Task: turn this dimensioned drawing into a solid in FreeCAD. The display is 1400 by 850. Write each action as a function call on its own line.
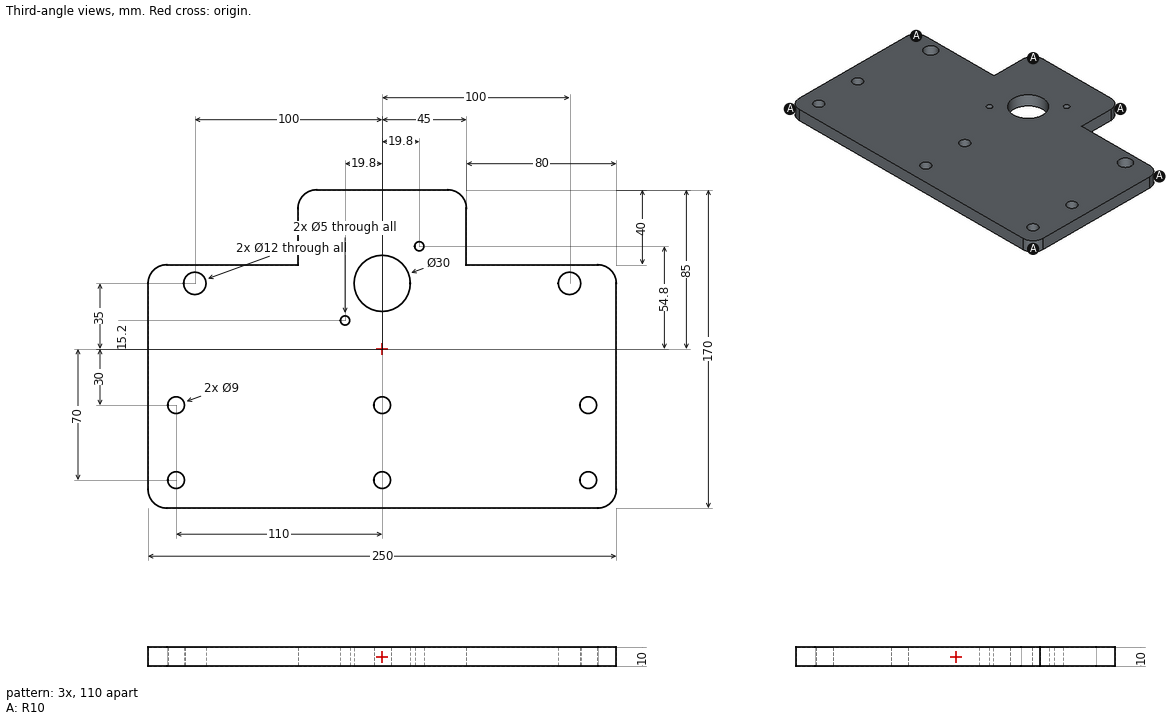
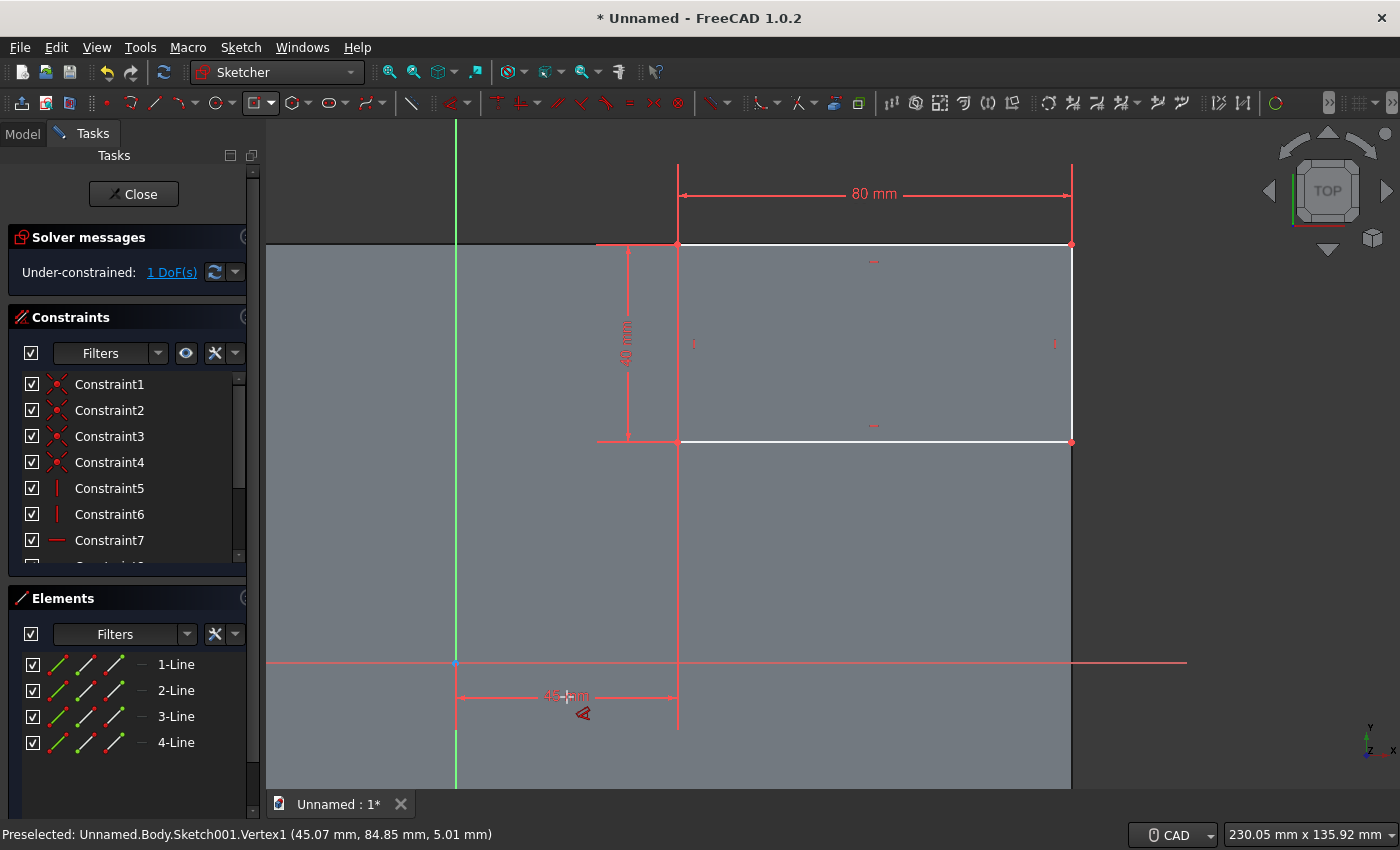
click(678, 245)
click(422, 454)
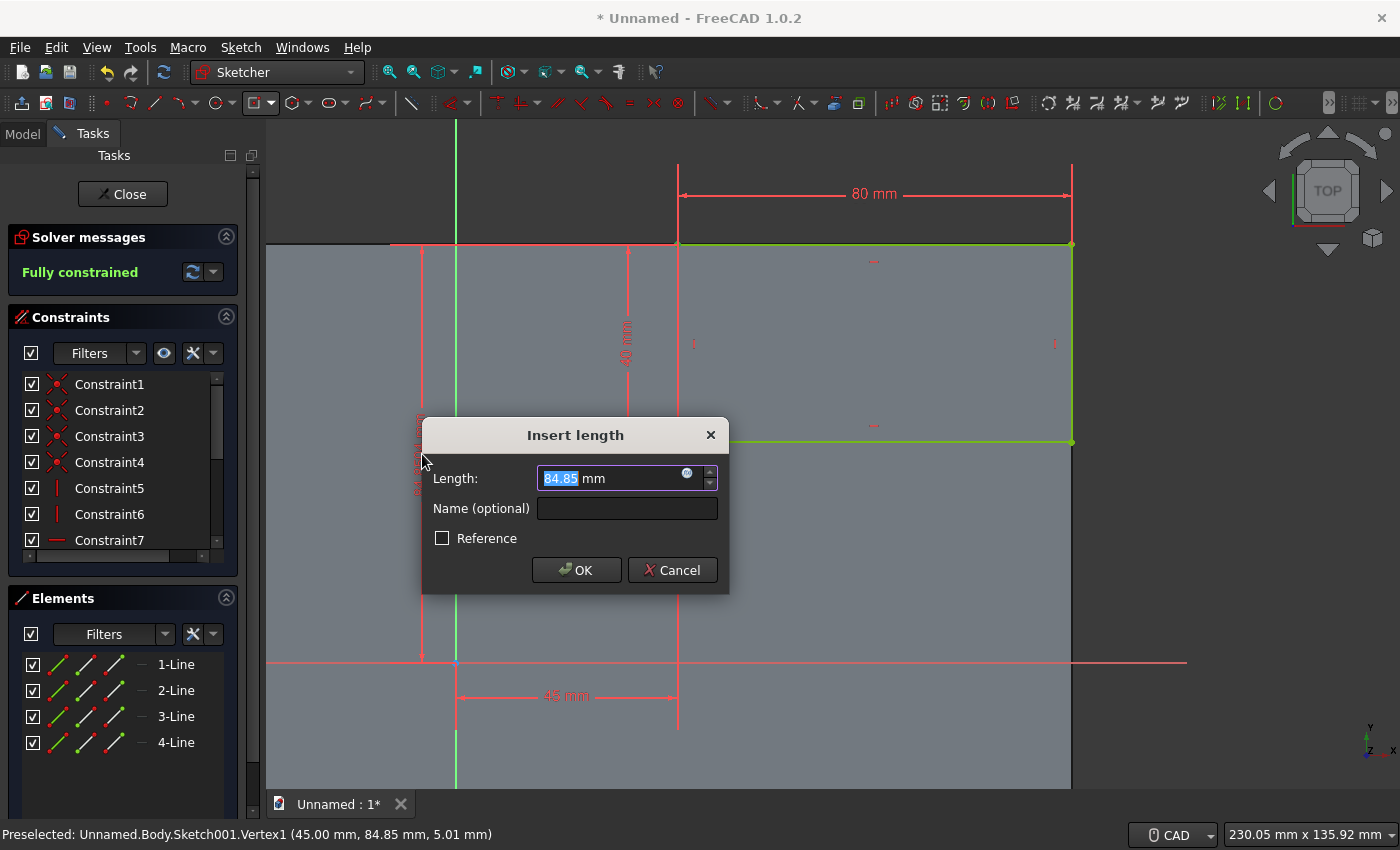
text(85)
key(Return)
key(Escape)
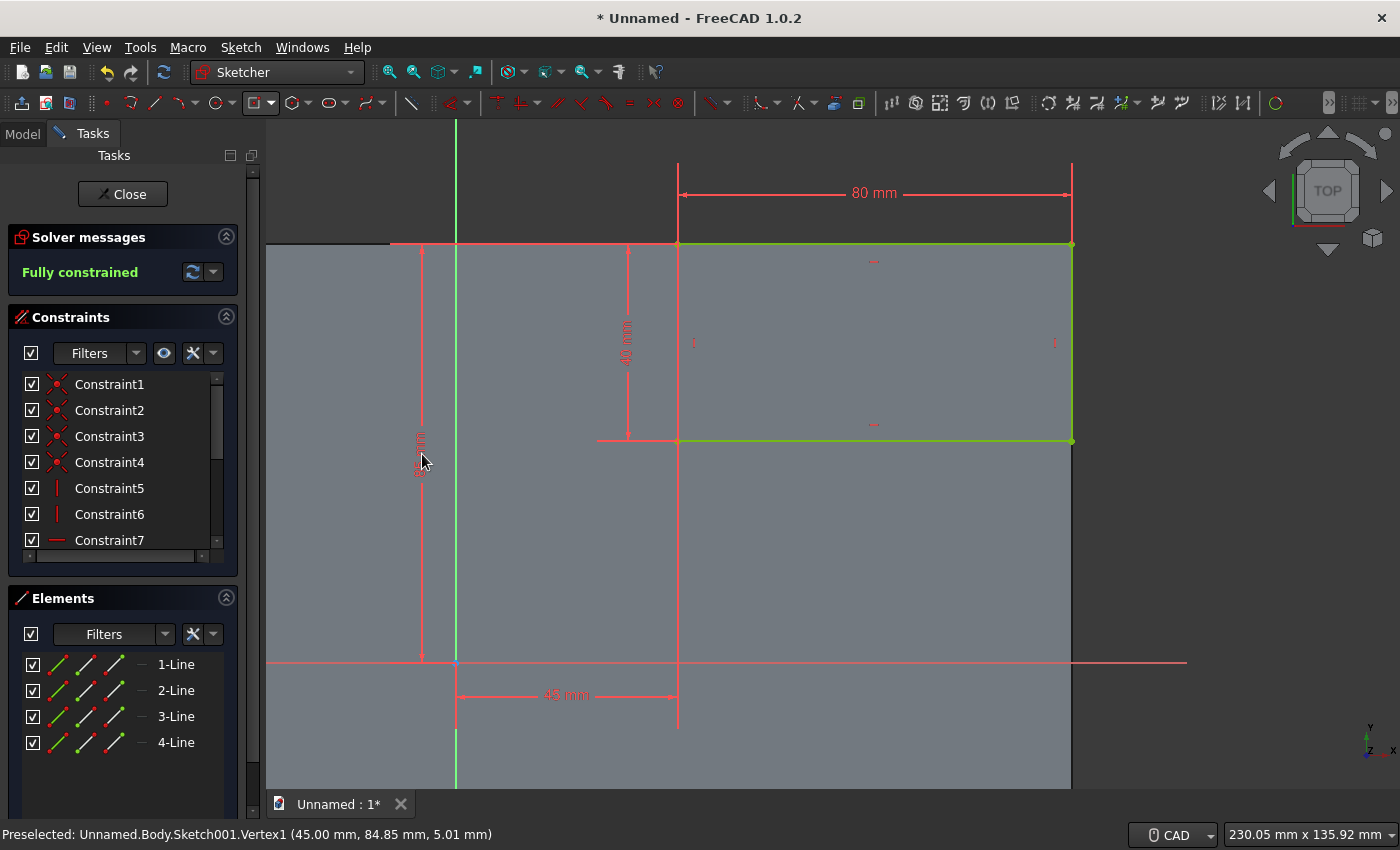
click(123, 194)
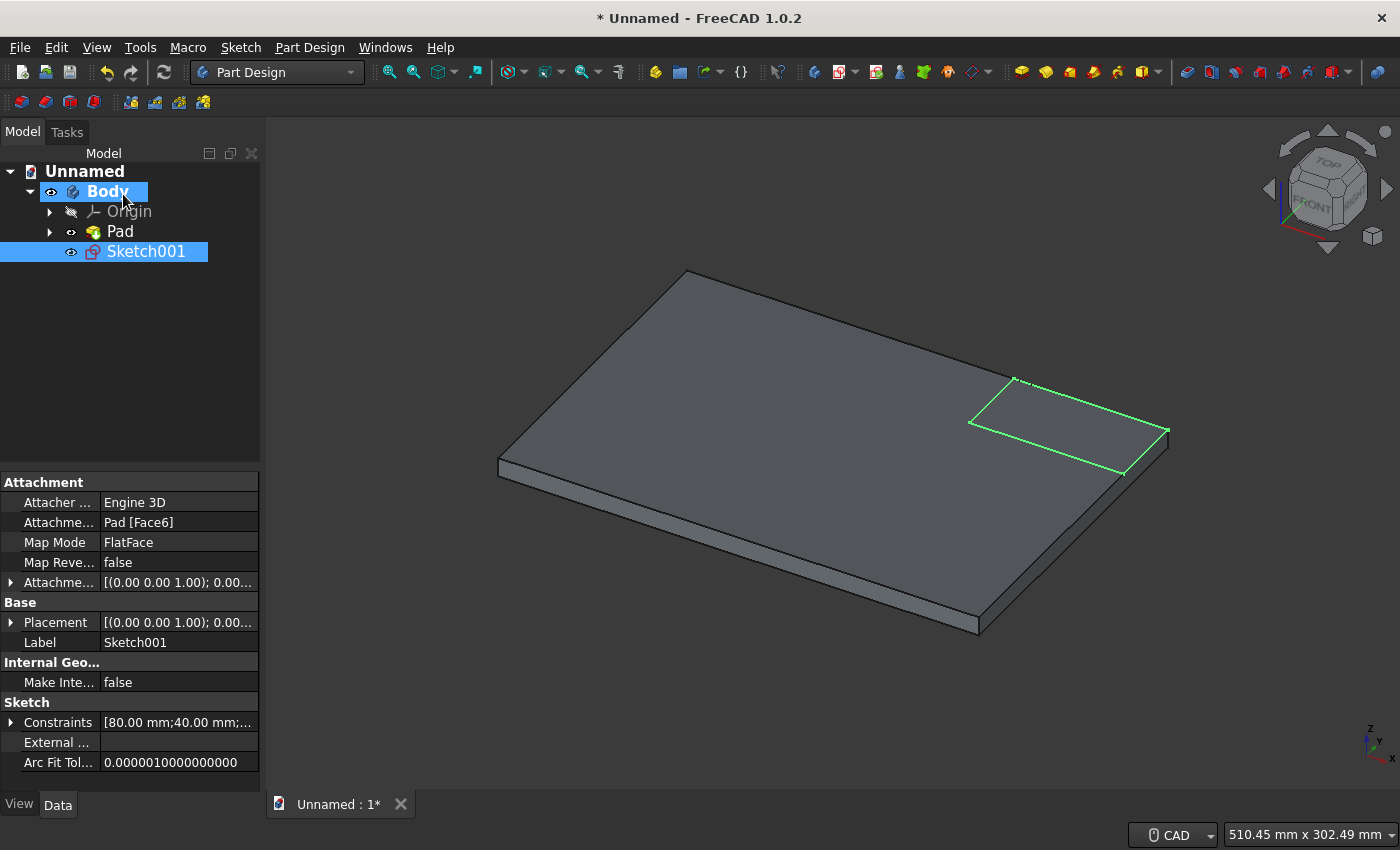
click(1188, 72)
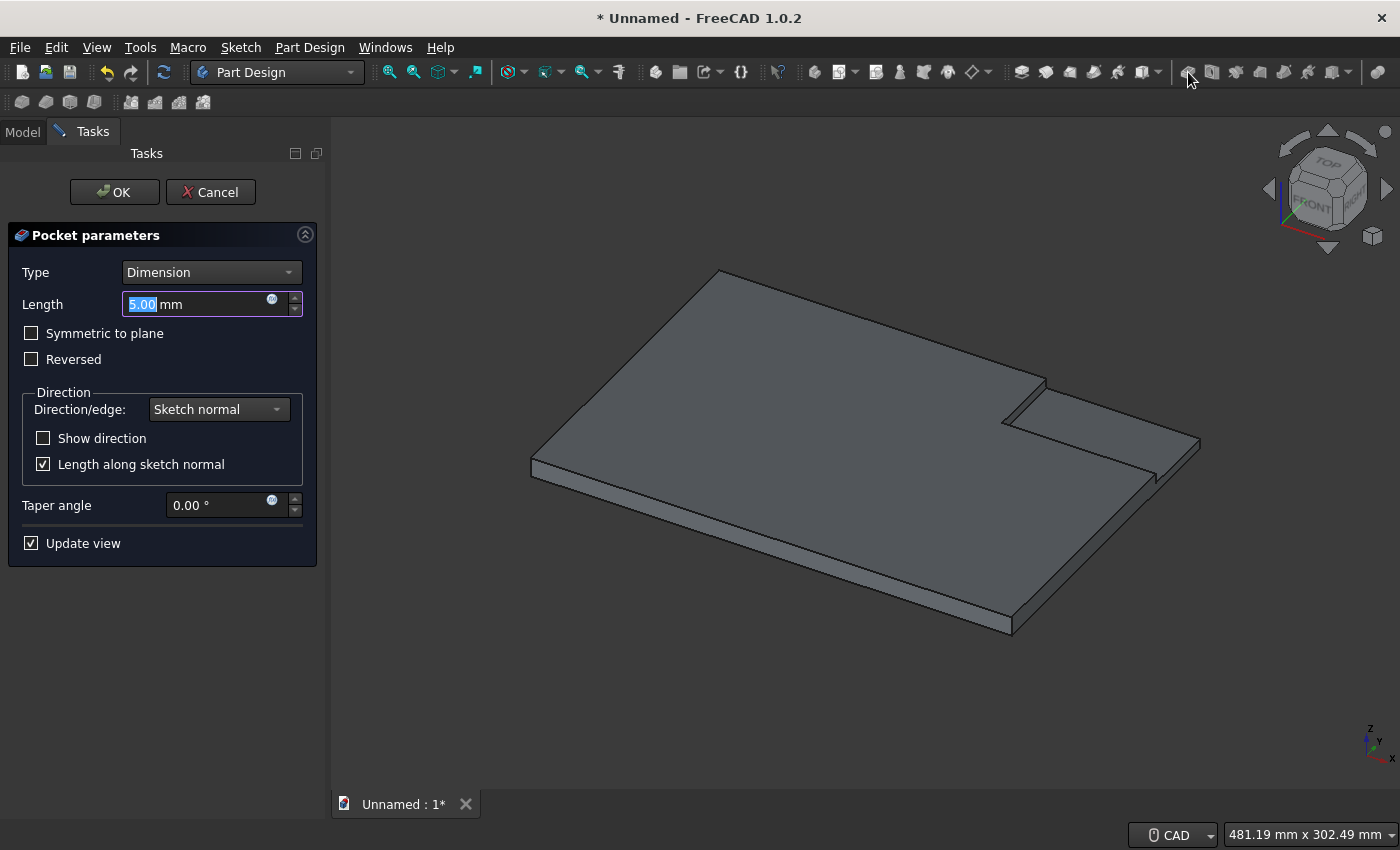
text(10)
key(Tab)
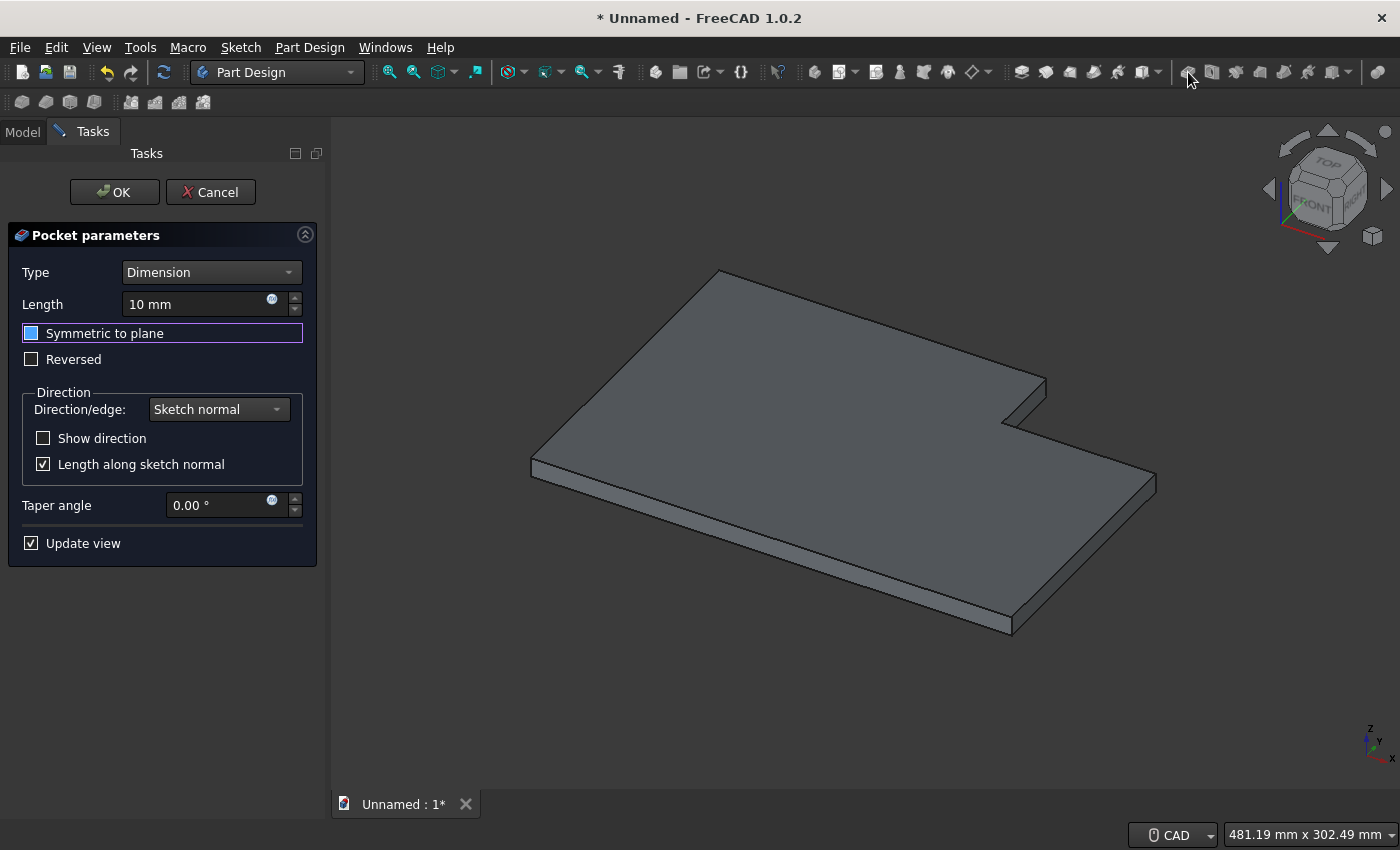
click(115, 192)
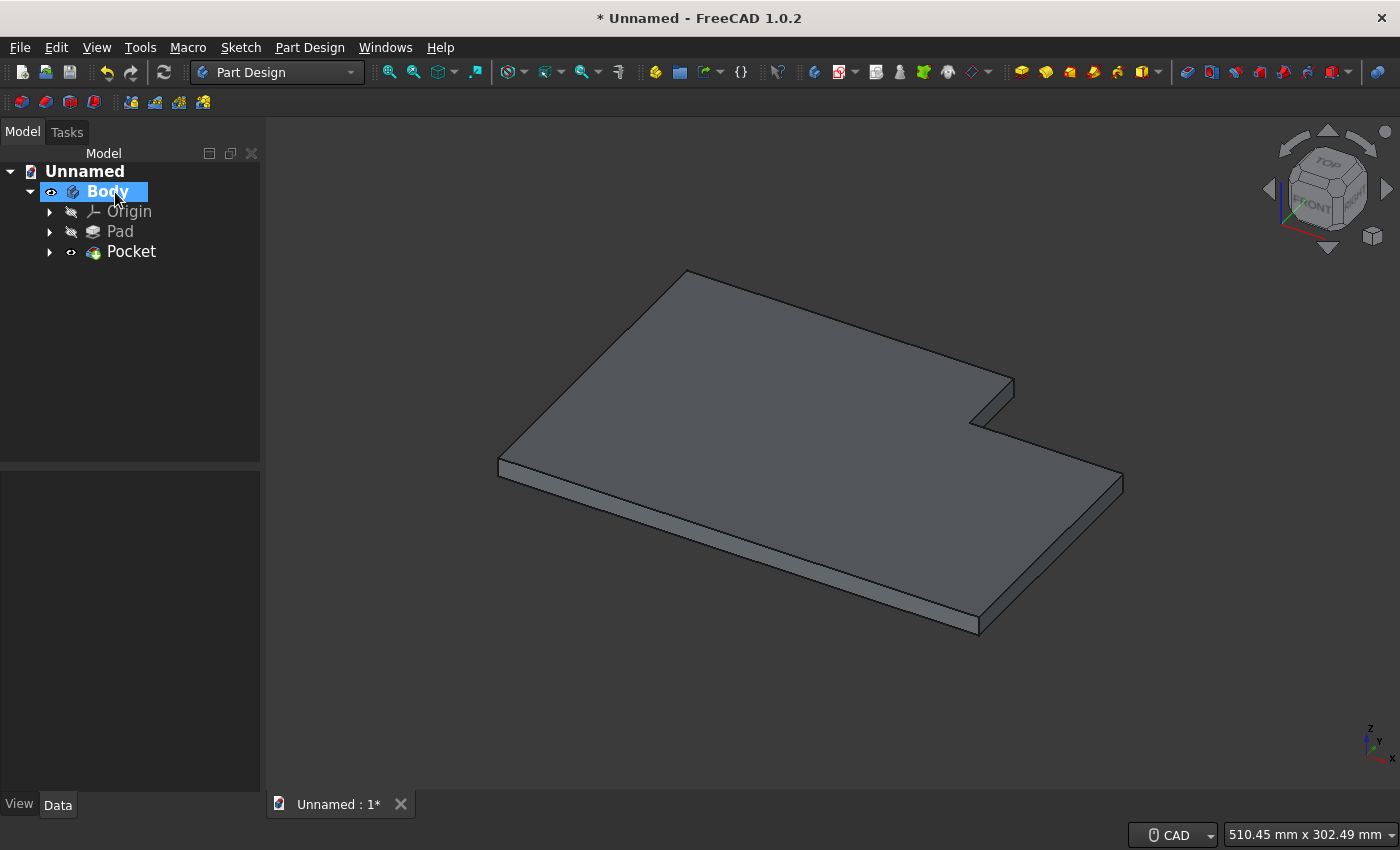
click(116, 252)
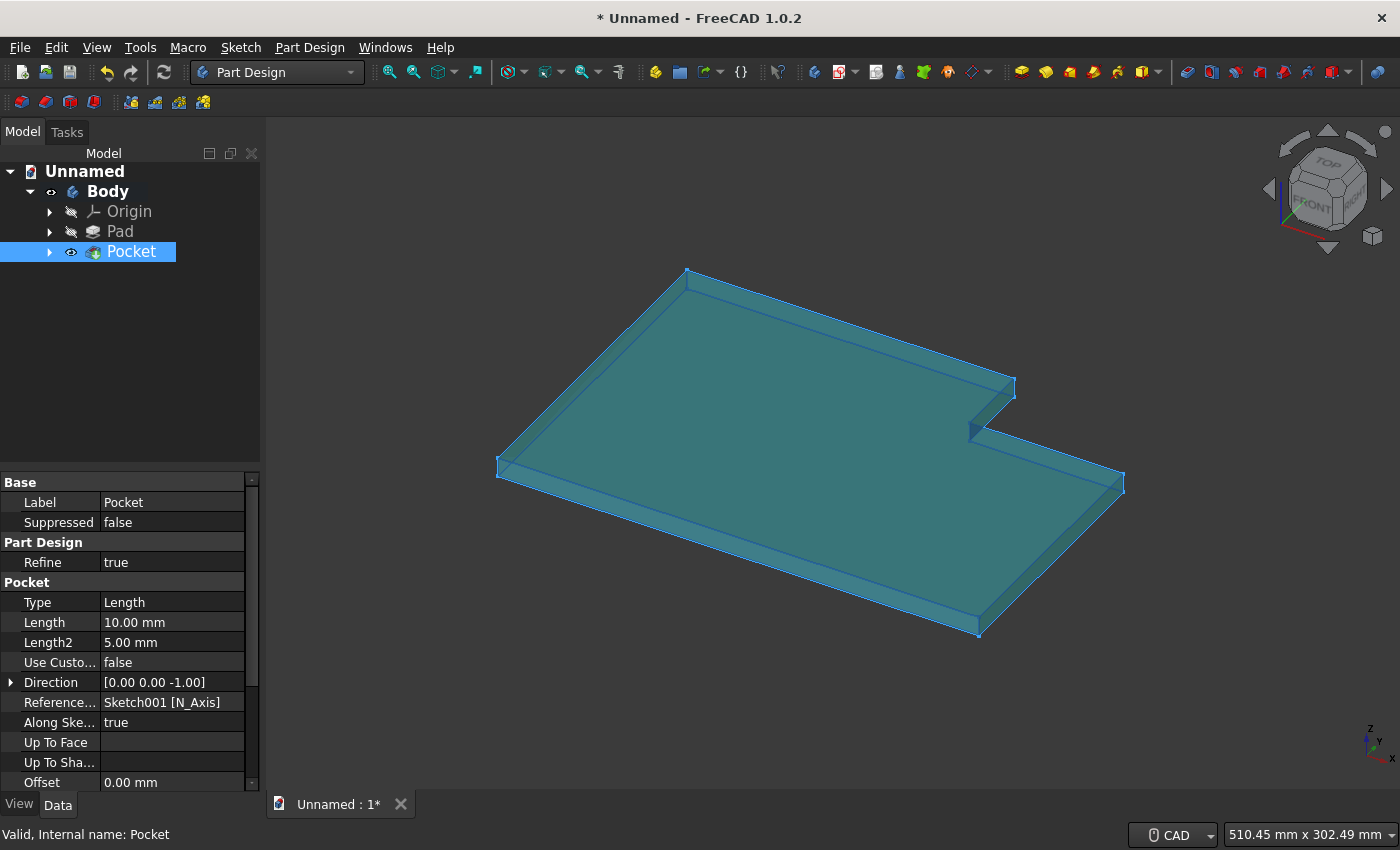
click(132, 102)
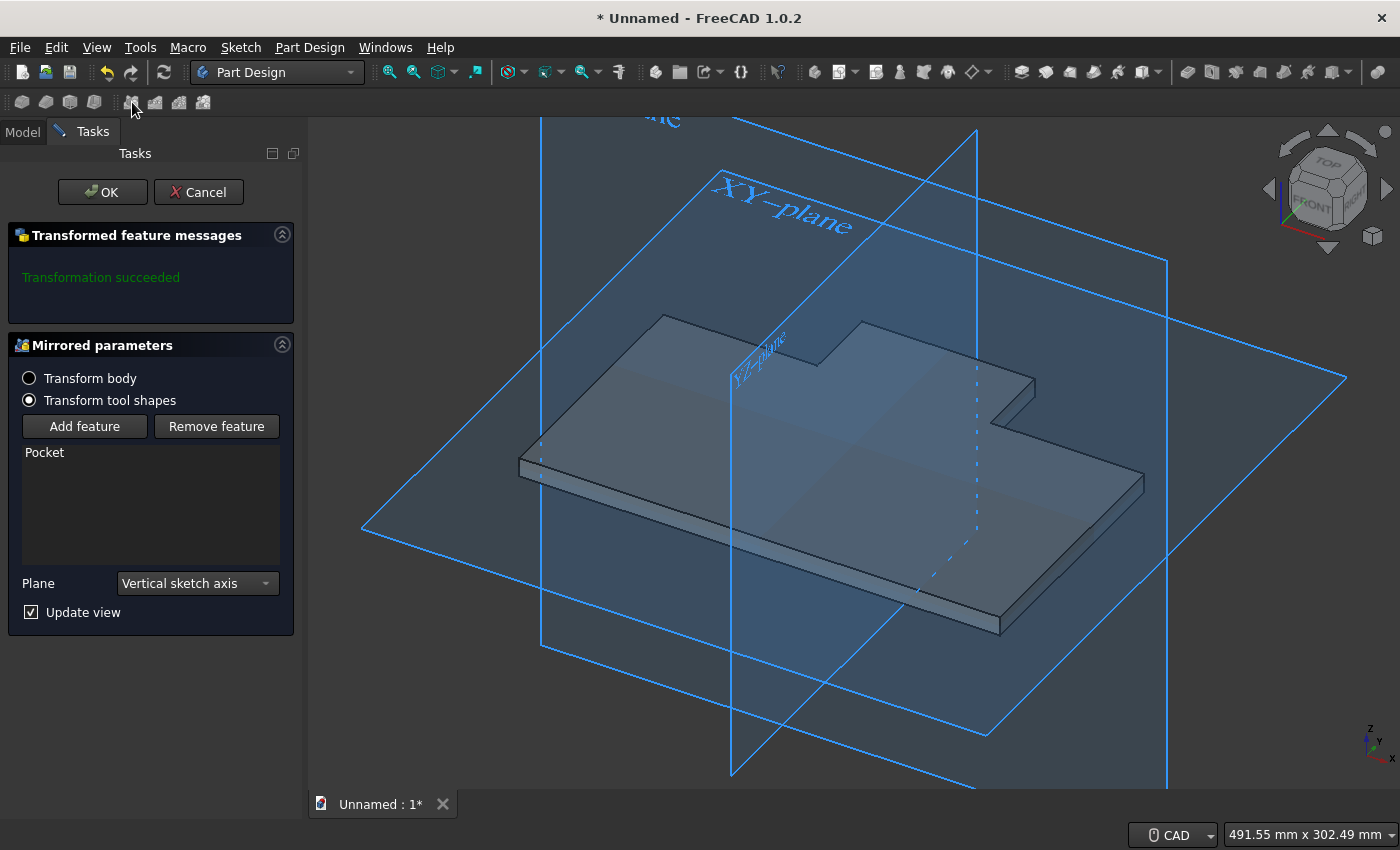
click(198, 584)